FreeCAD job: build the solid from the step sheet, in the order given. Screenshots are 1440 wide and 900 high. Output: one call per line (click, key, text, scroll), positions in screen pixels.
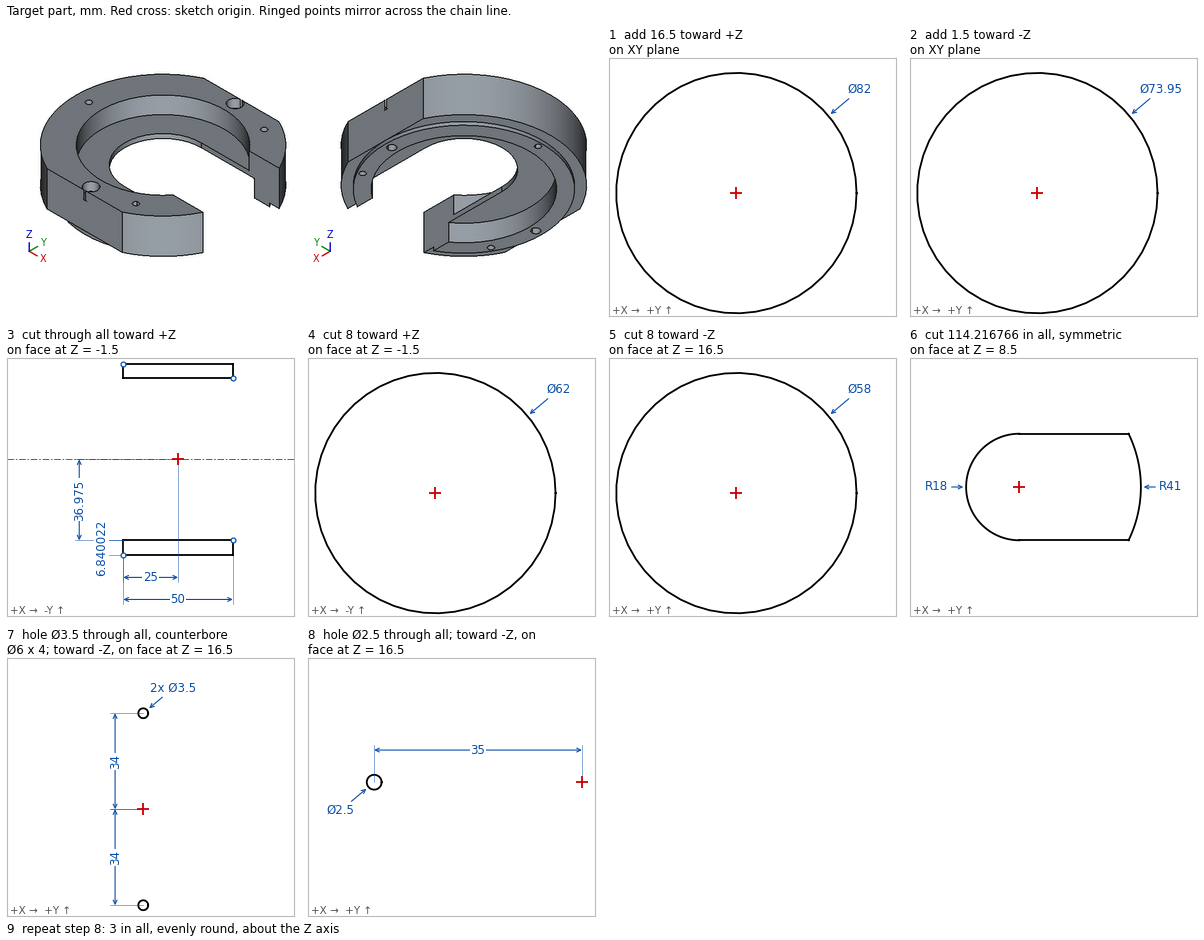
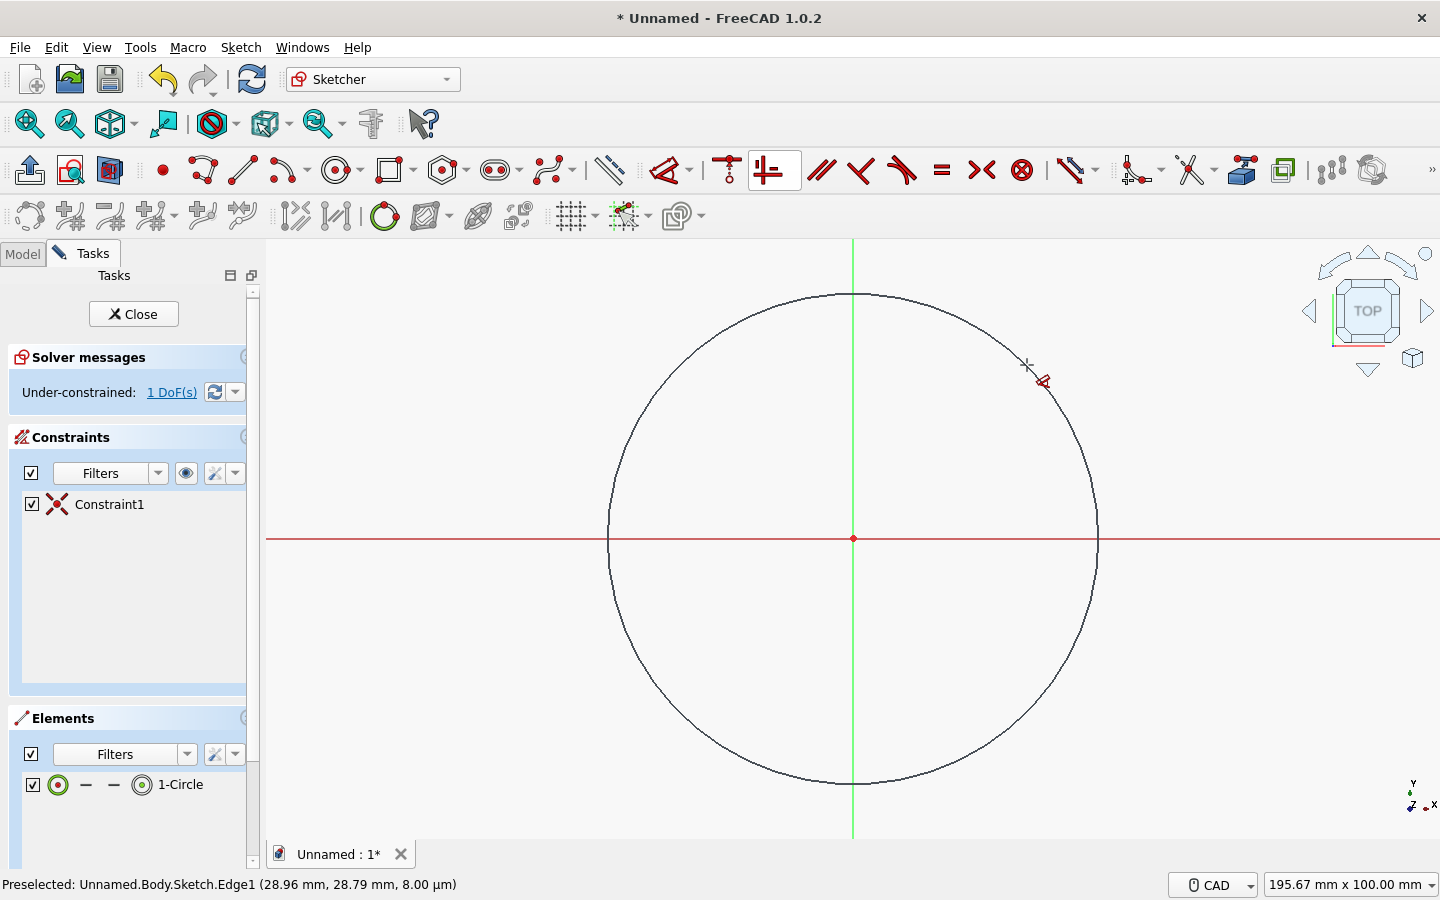
click(1026, 365)
click(1049, 342)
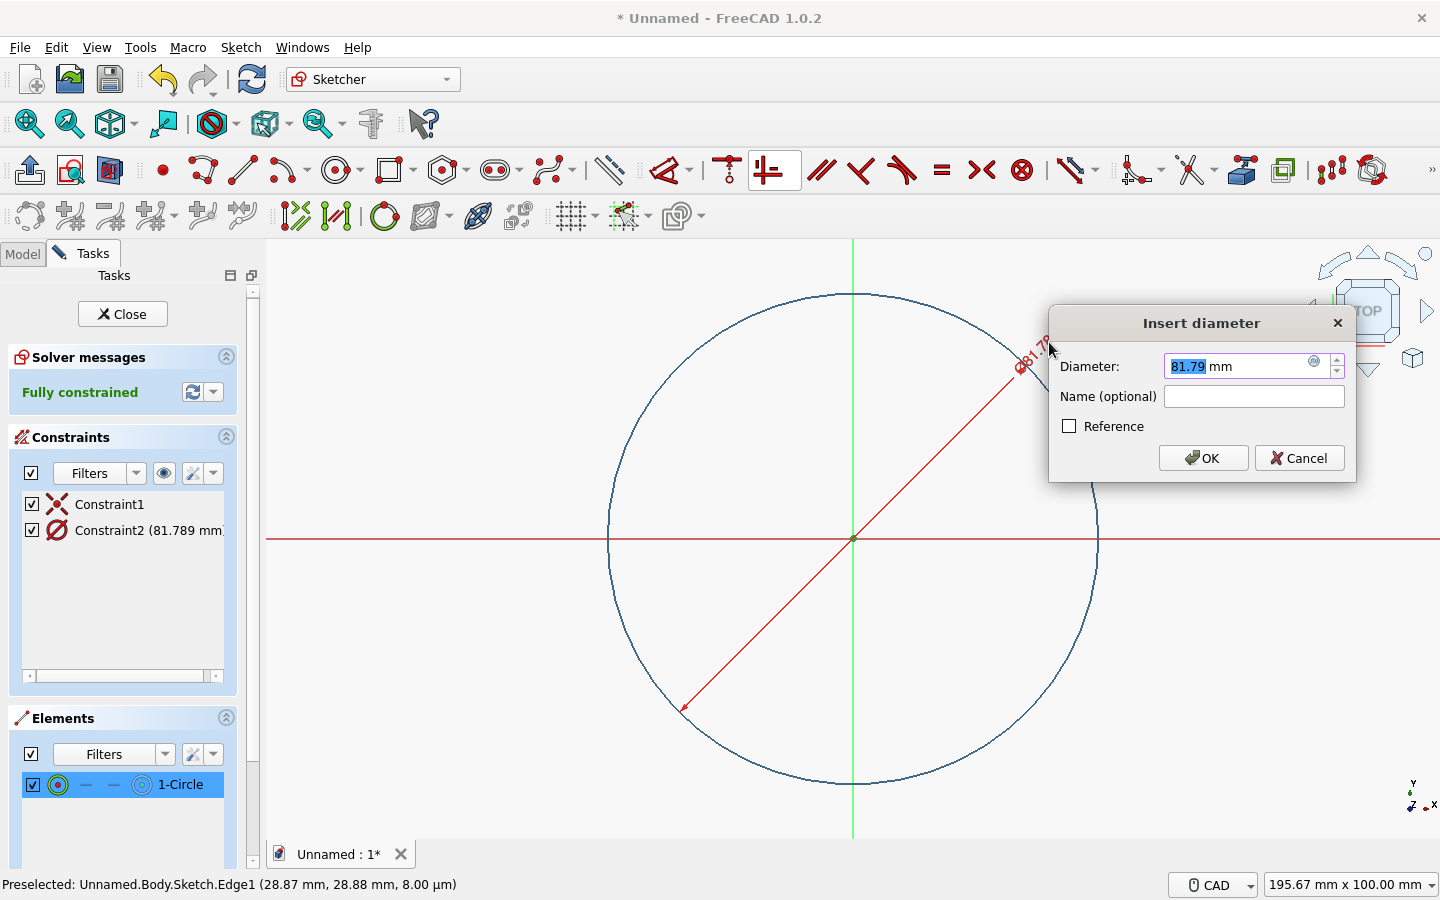
text(82)
key(Return)
key(Escape)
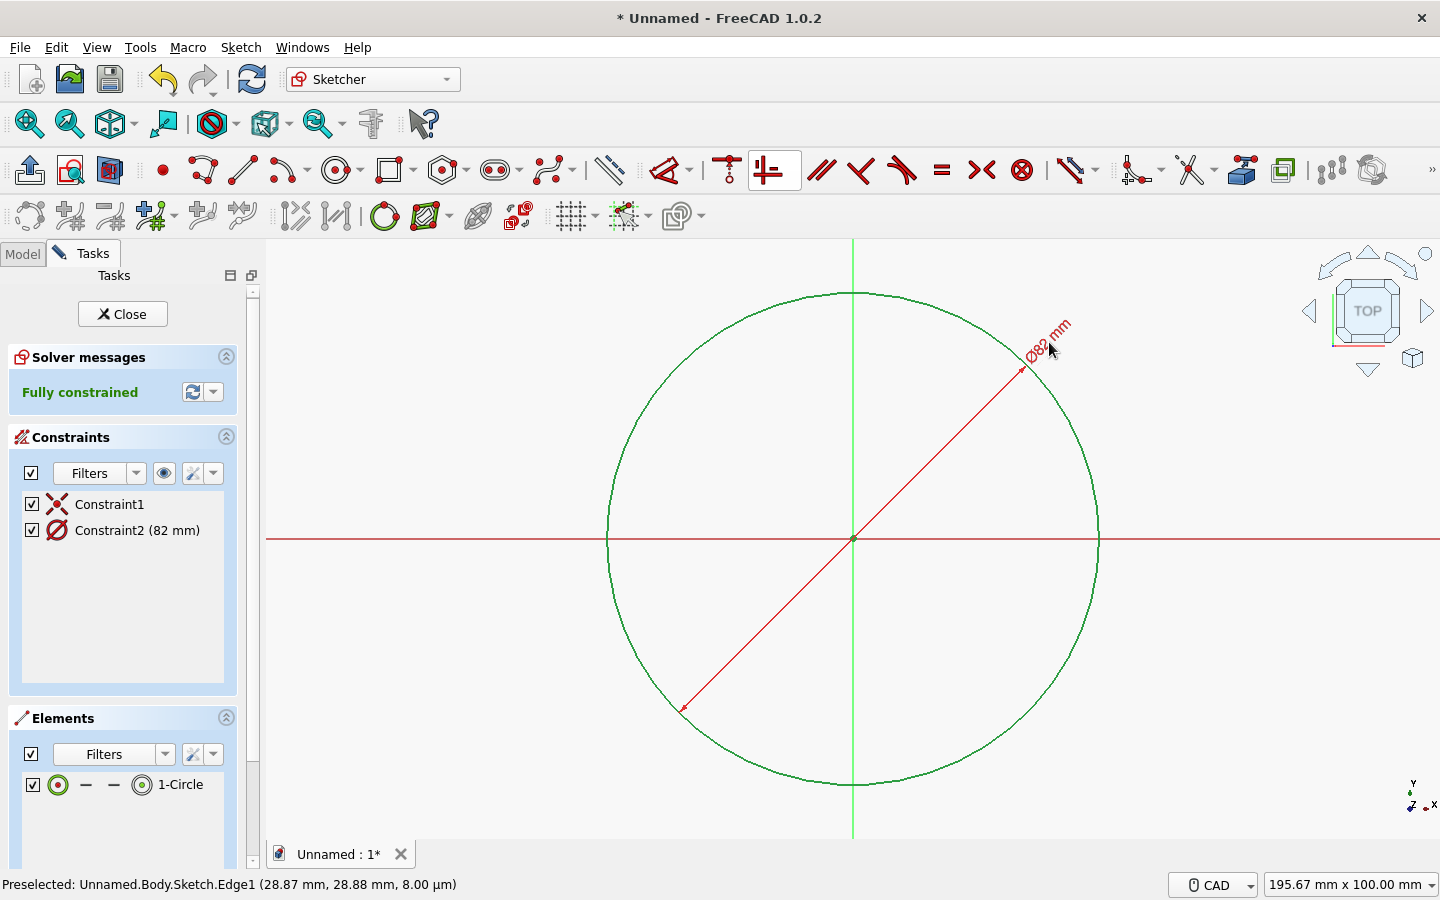
click(123, 314)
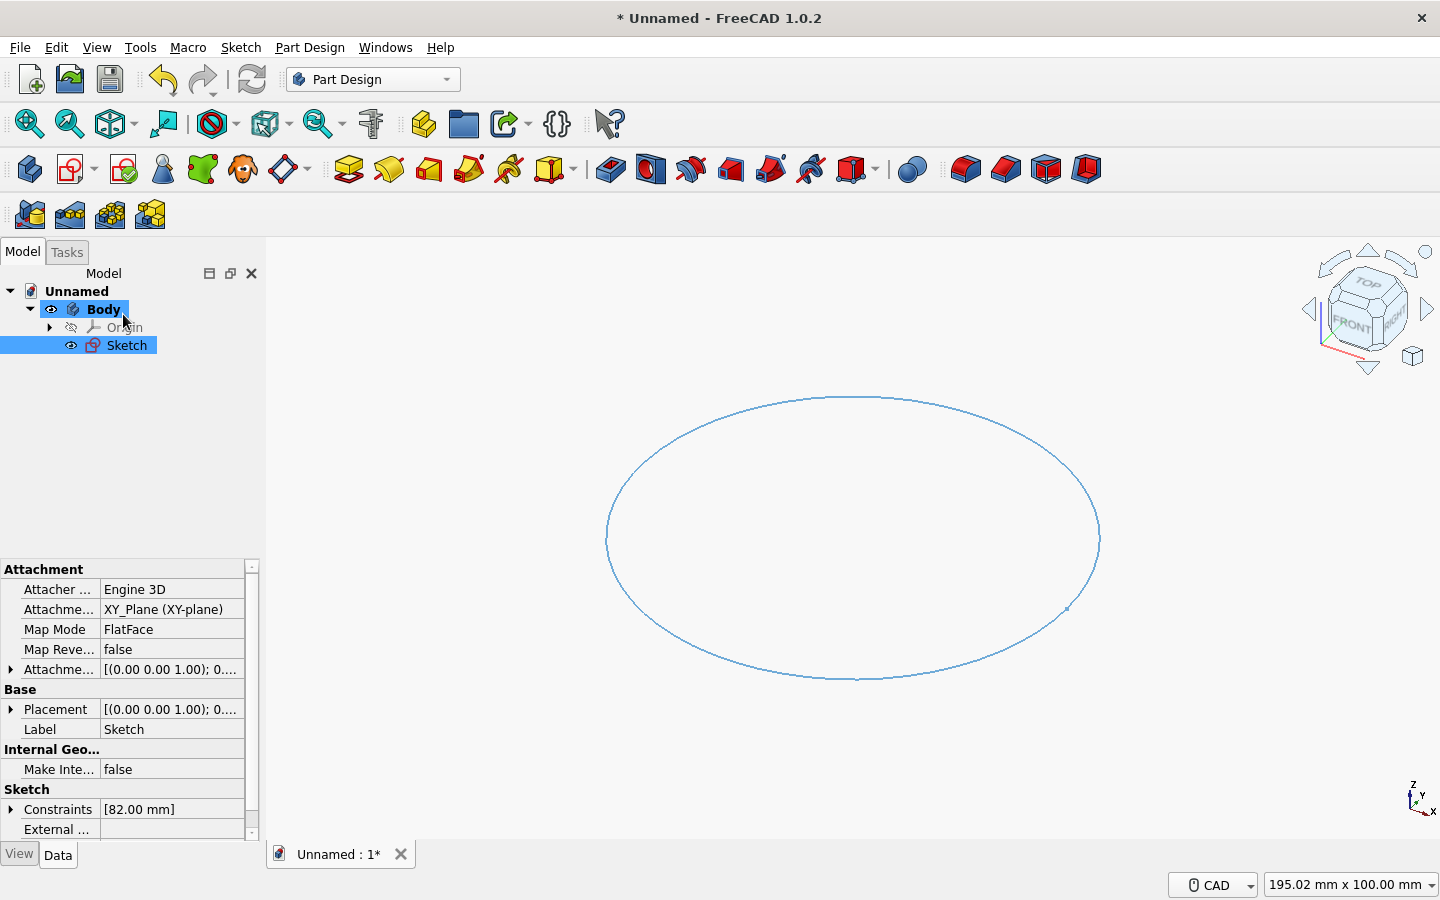
click(350, 170)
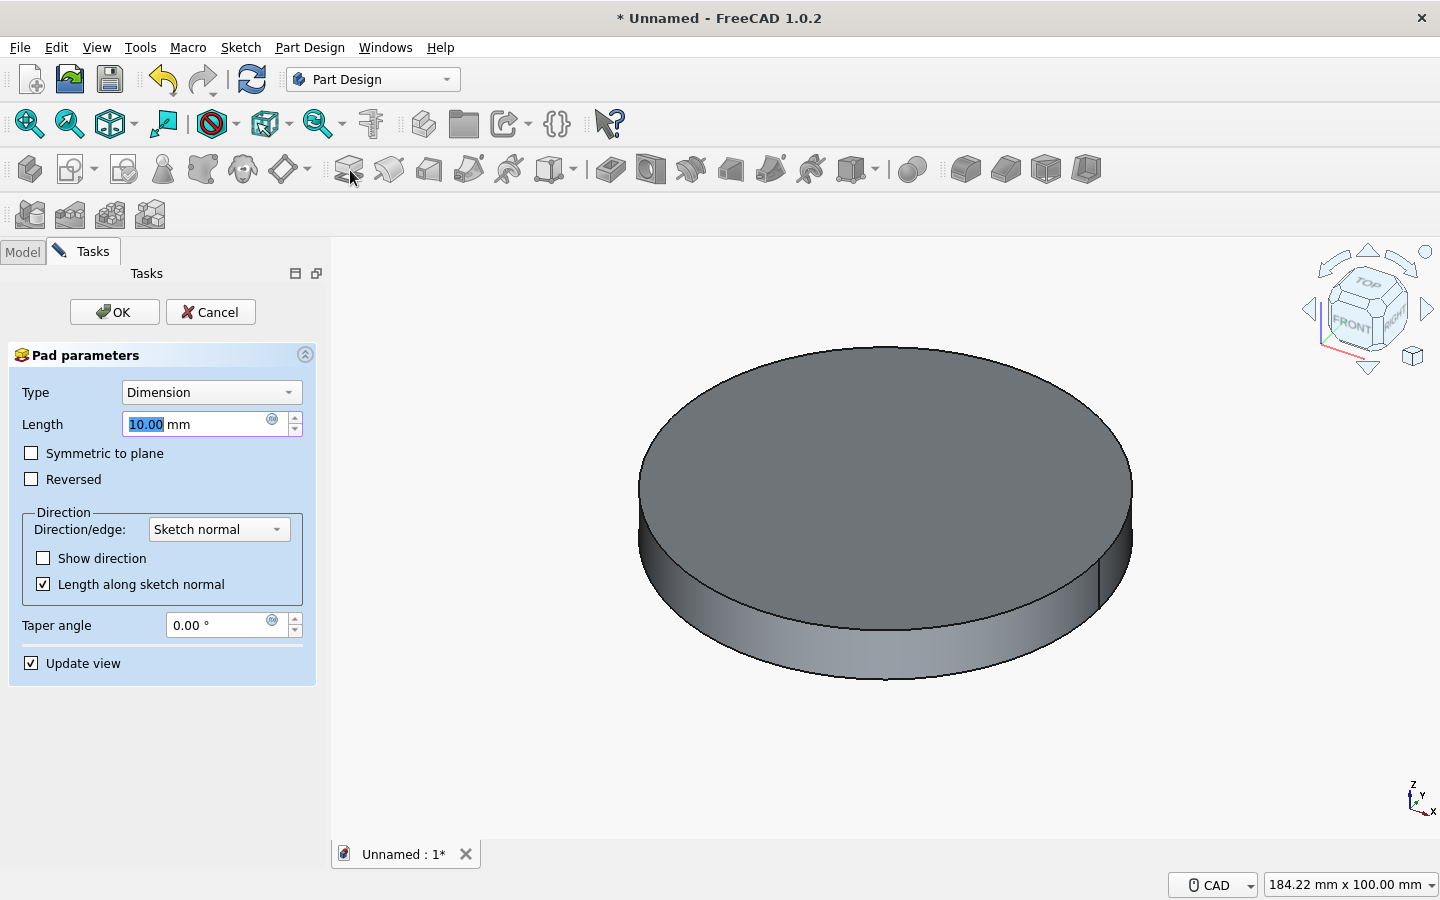
text(16.5)
key(Tab)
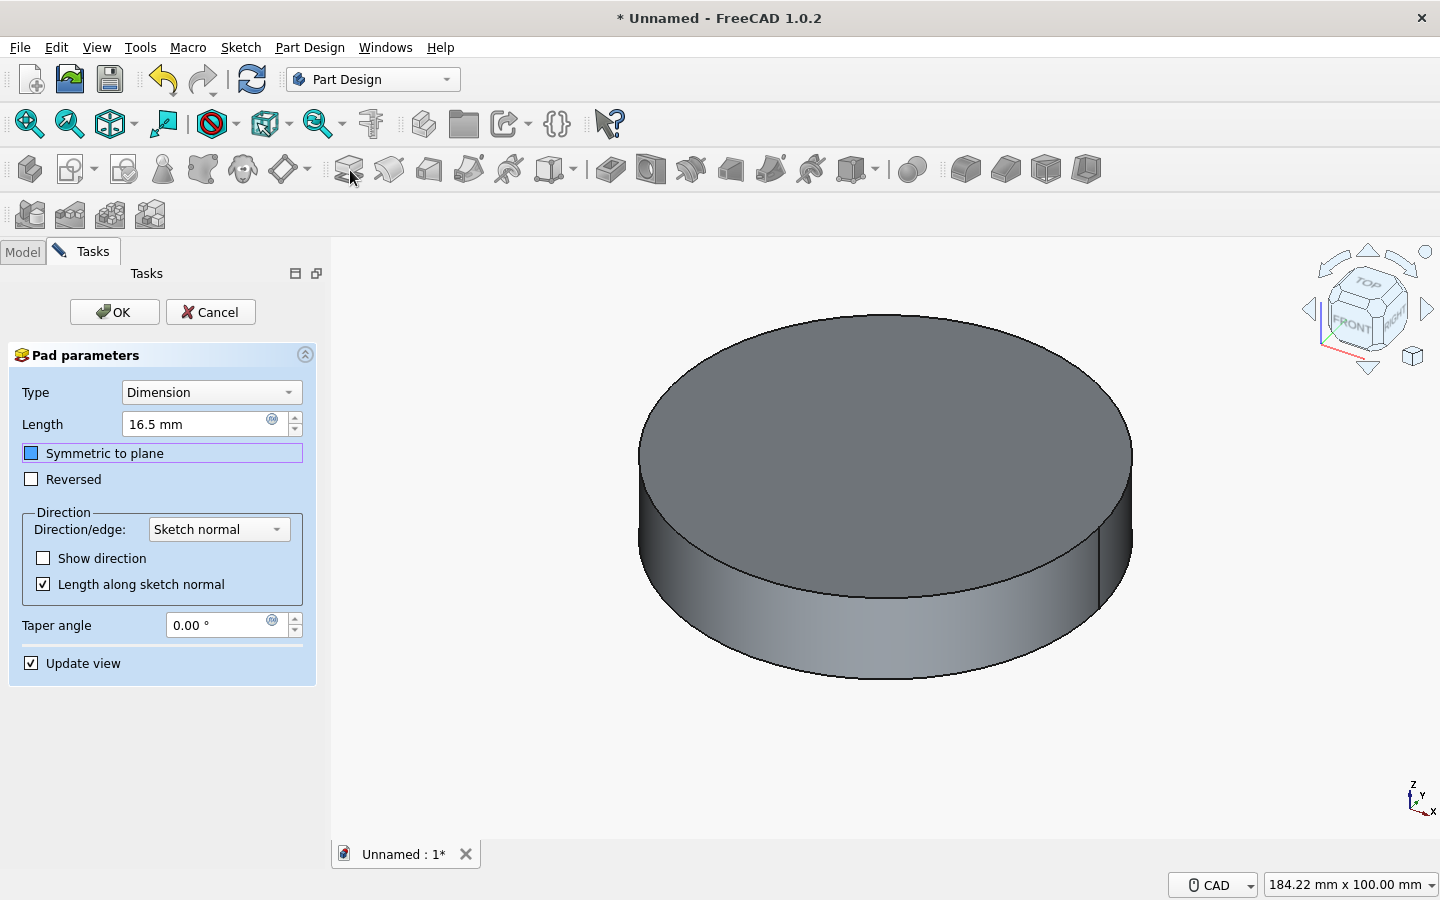
click(115, 312)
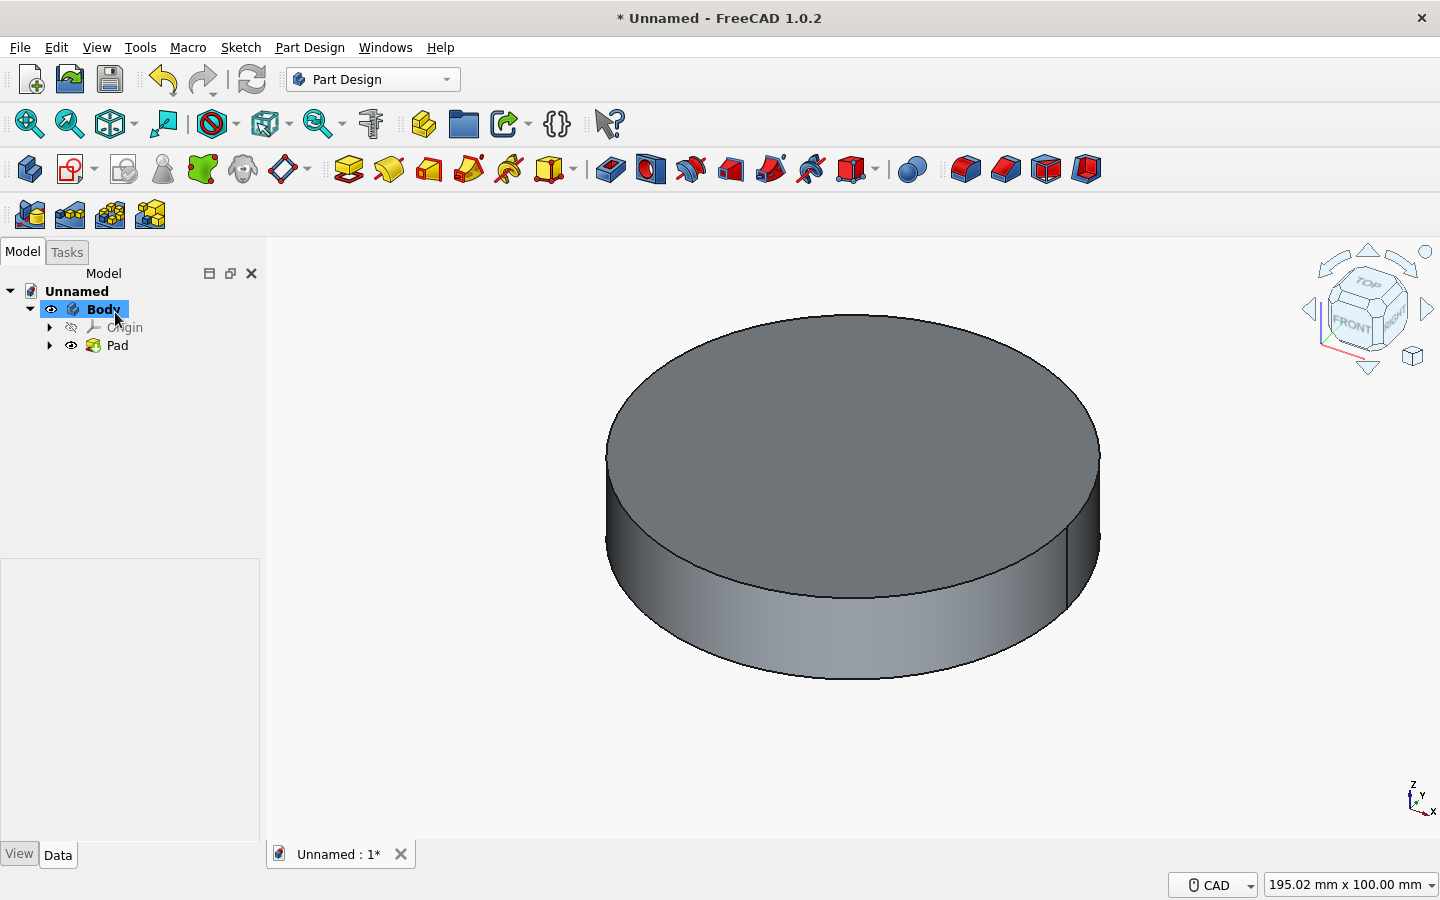
click(70, 170)